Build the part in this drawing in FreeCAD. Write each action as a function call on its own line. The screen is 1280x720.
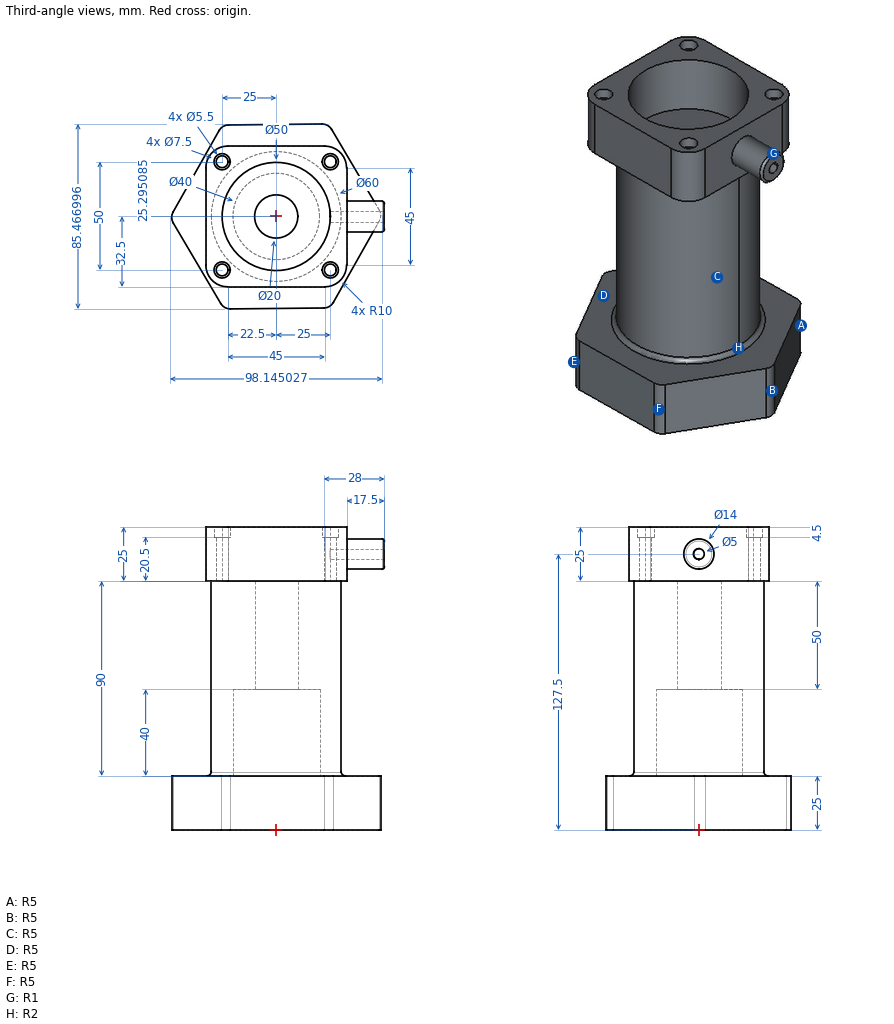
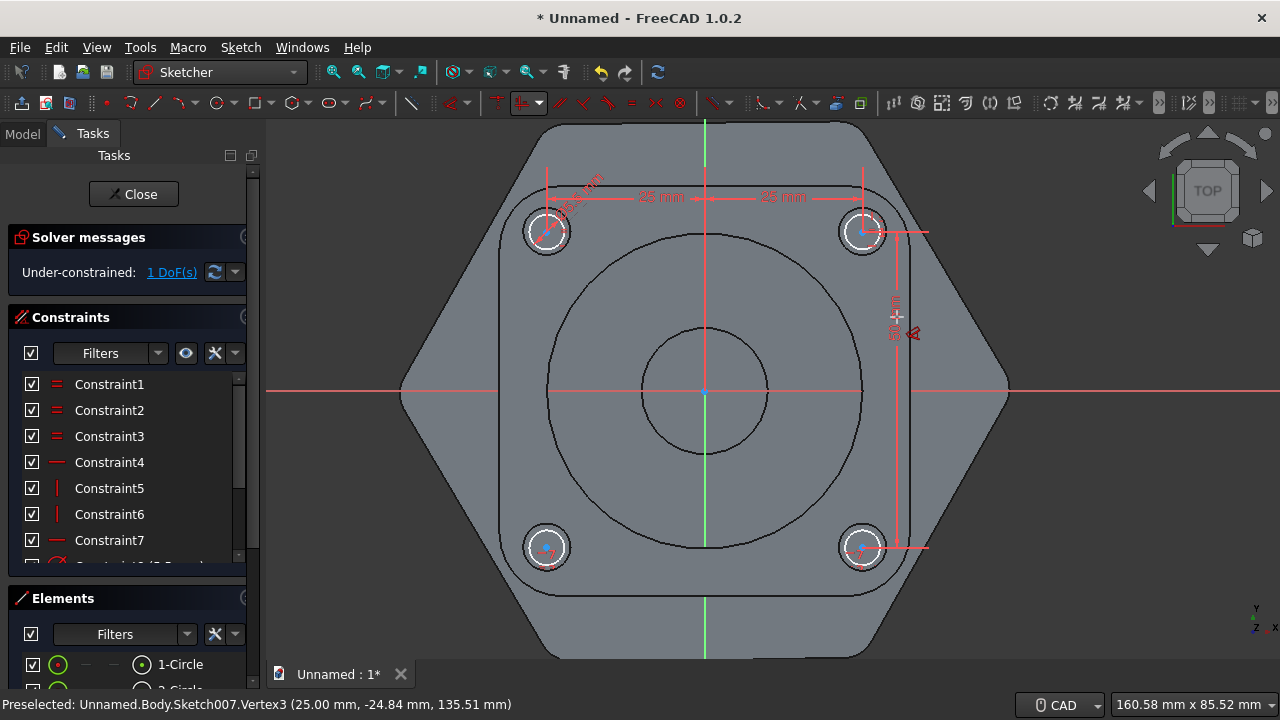
click(547, 232)
click(513, 312)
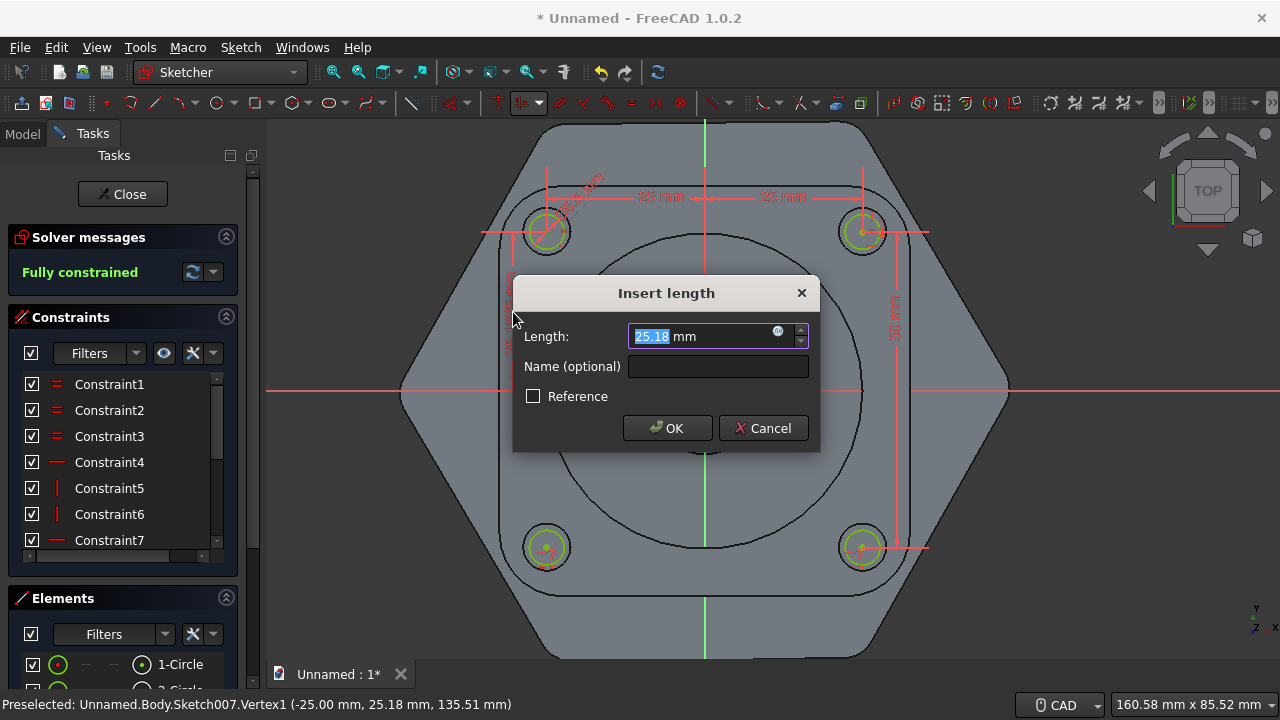
text(25.295085)
key(Return)
key(Escape)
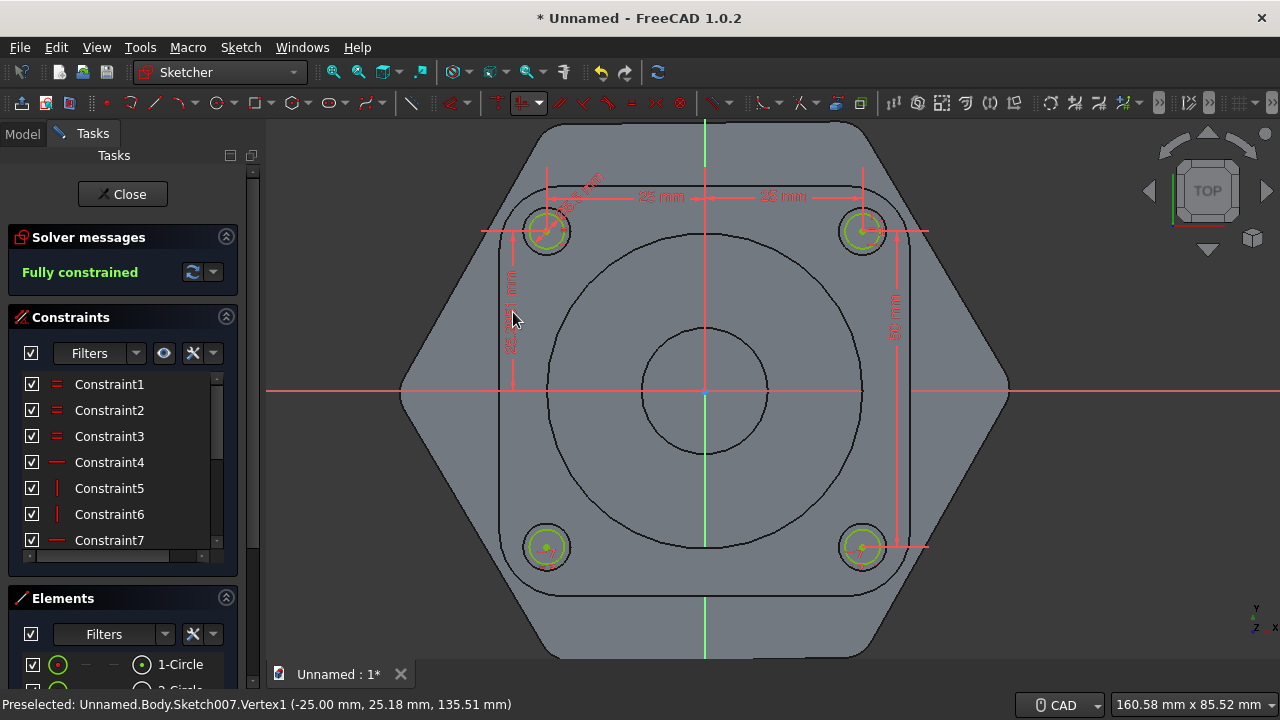
click(123, 194)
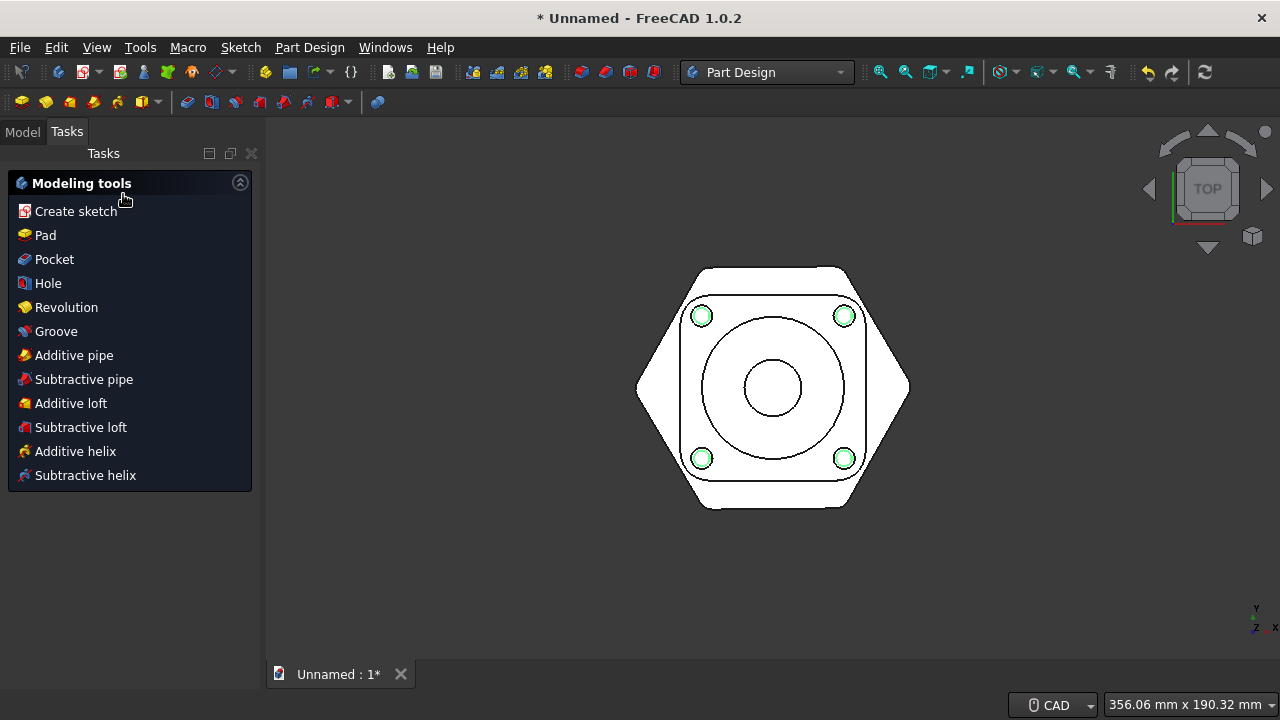
click(188, 102)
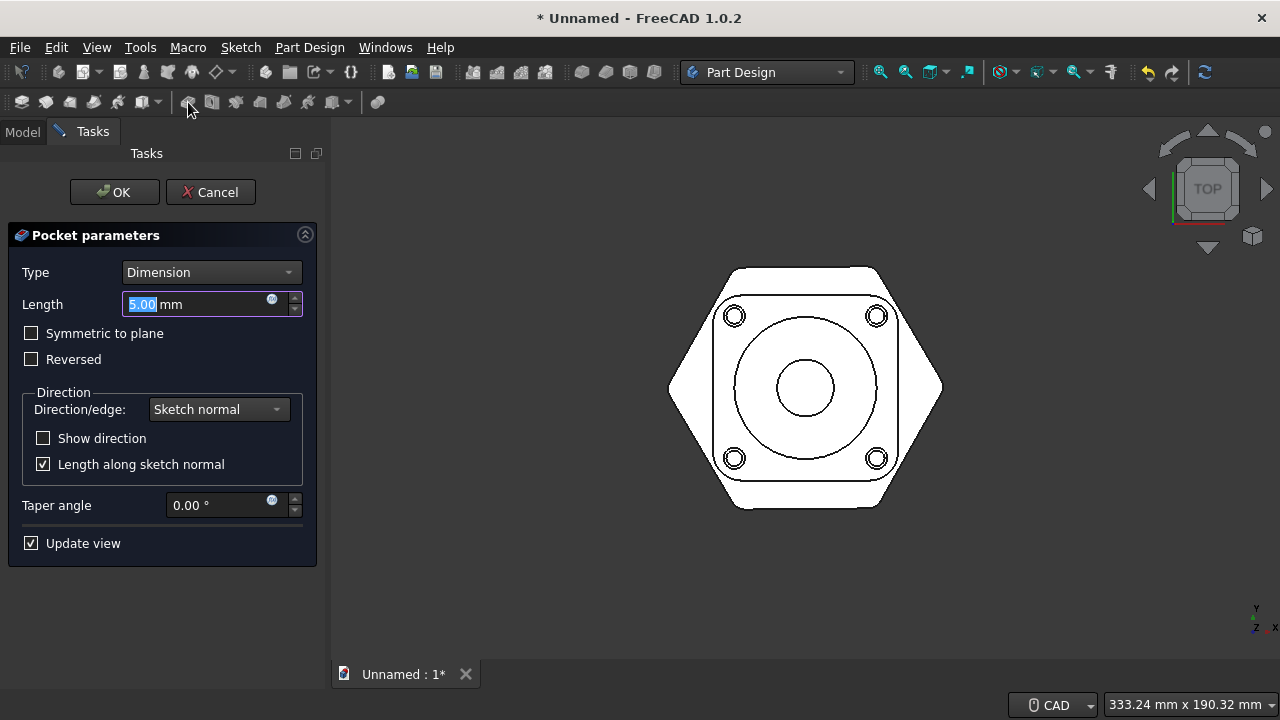
text(20.5)
key(Tab)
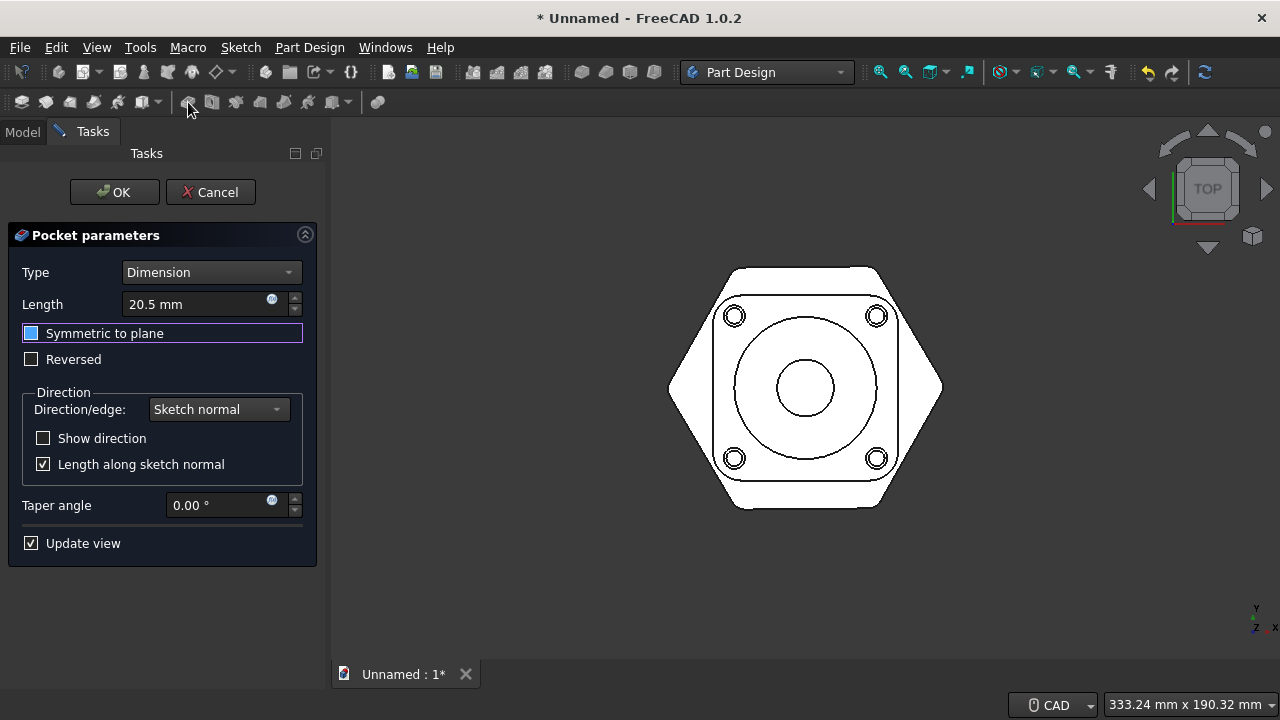
click(115, 192)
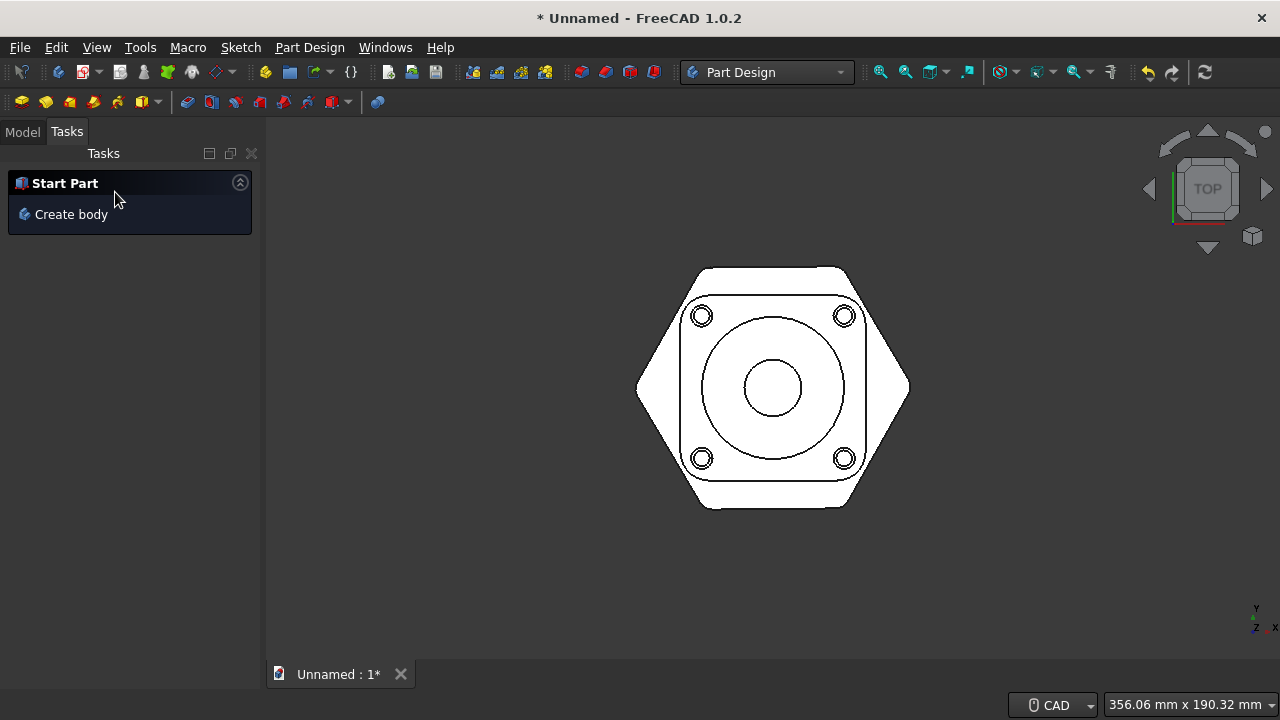
key(0)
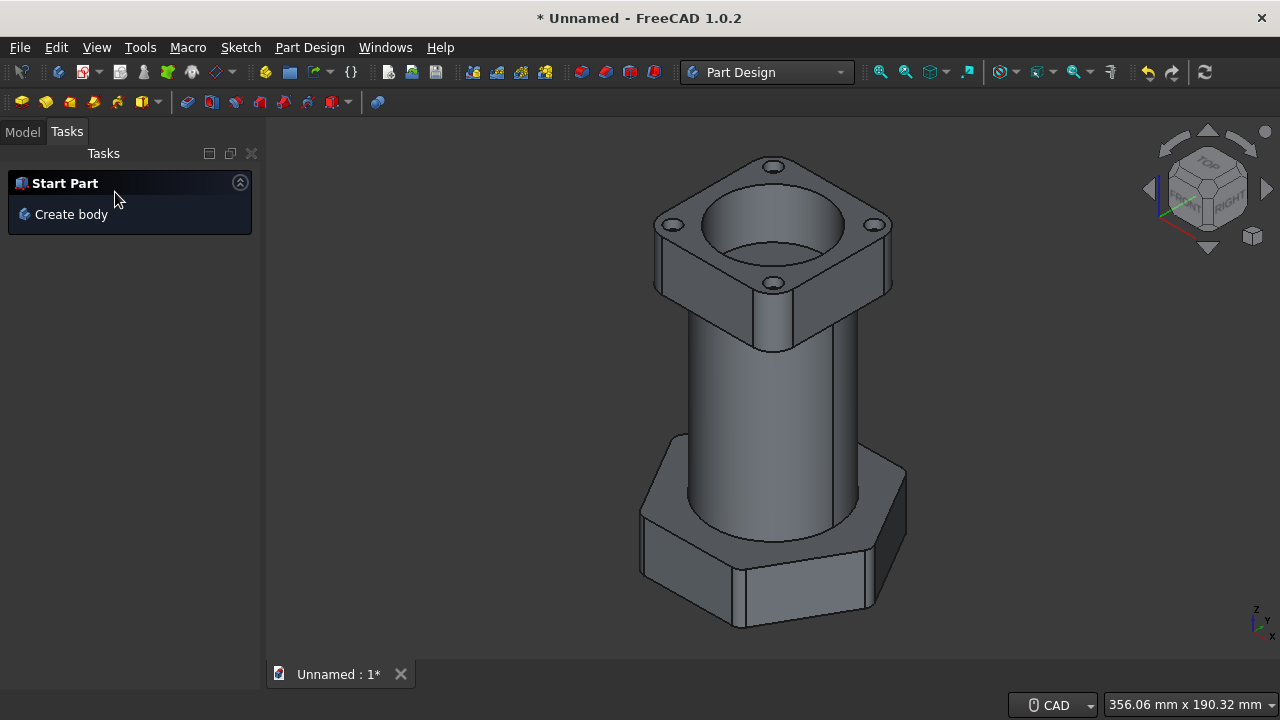
click(851, 284)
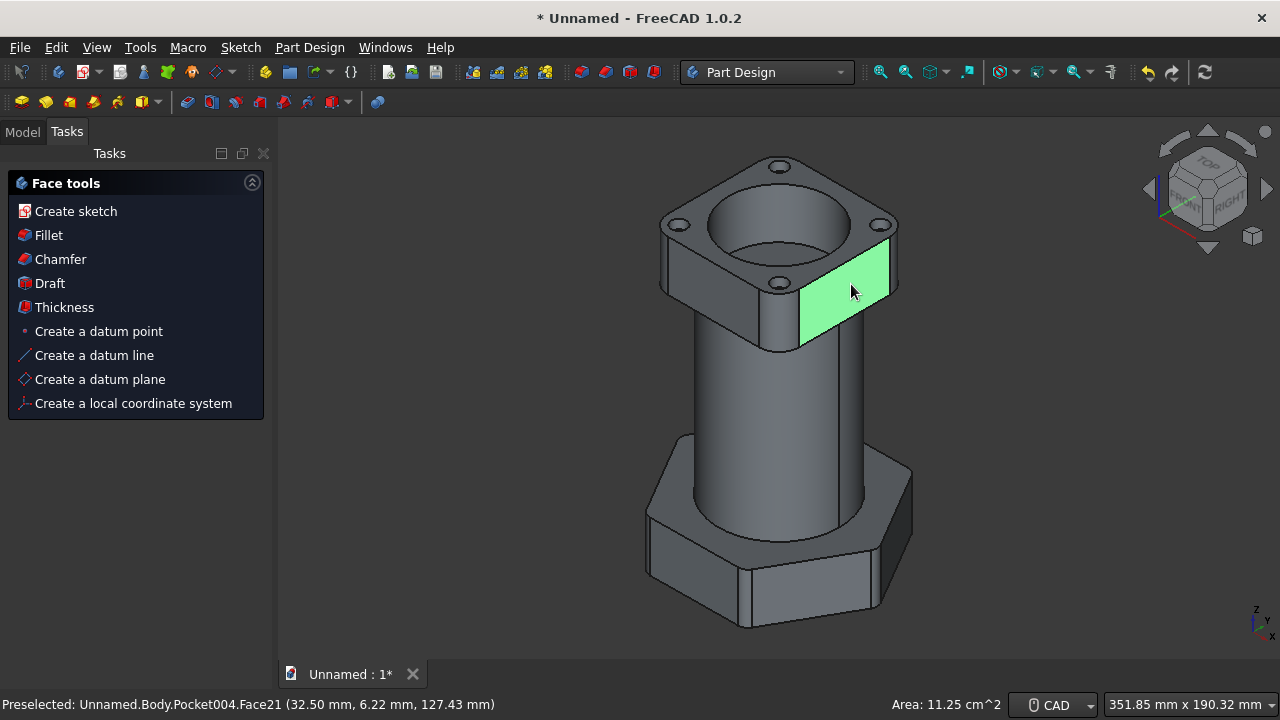
click(84, 72)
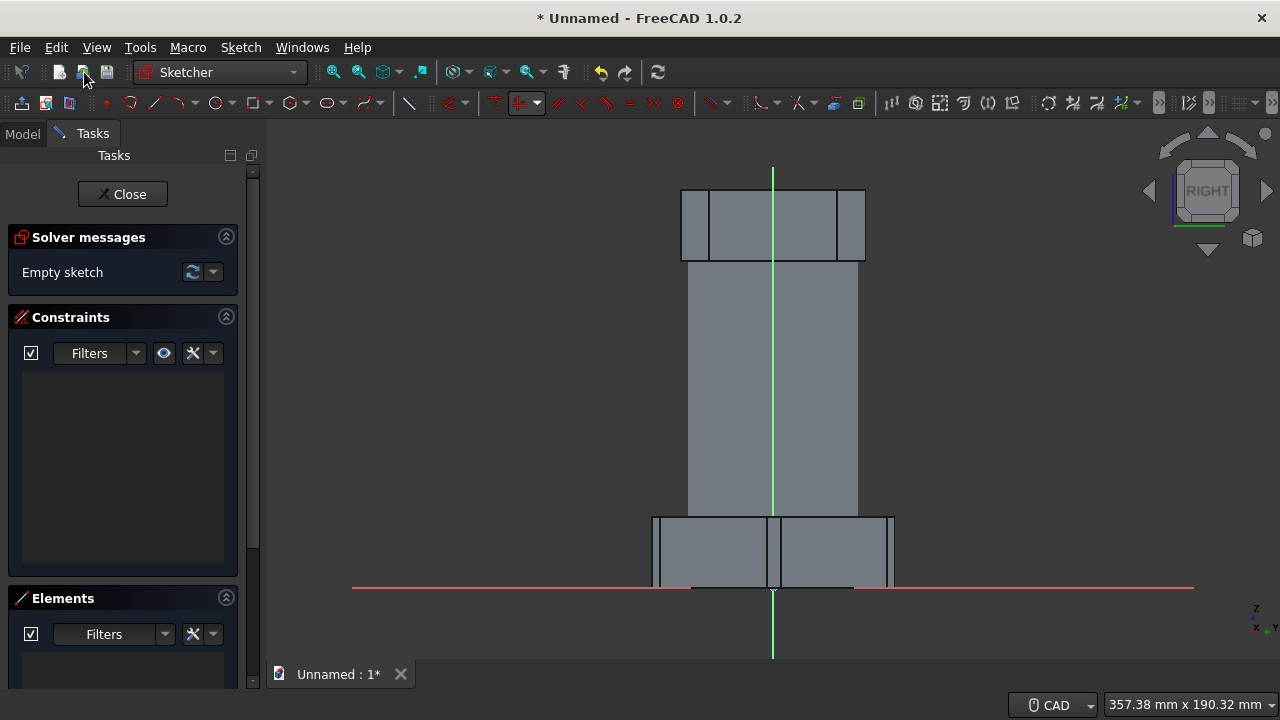
scroll(782, 206, up, 11)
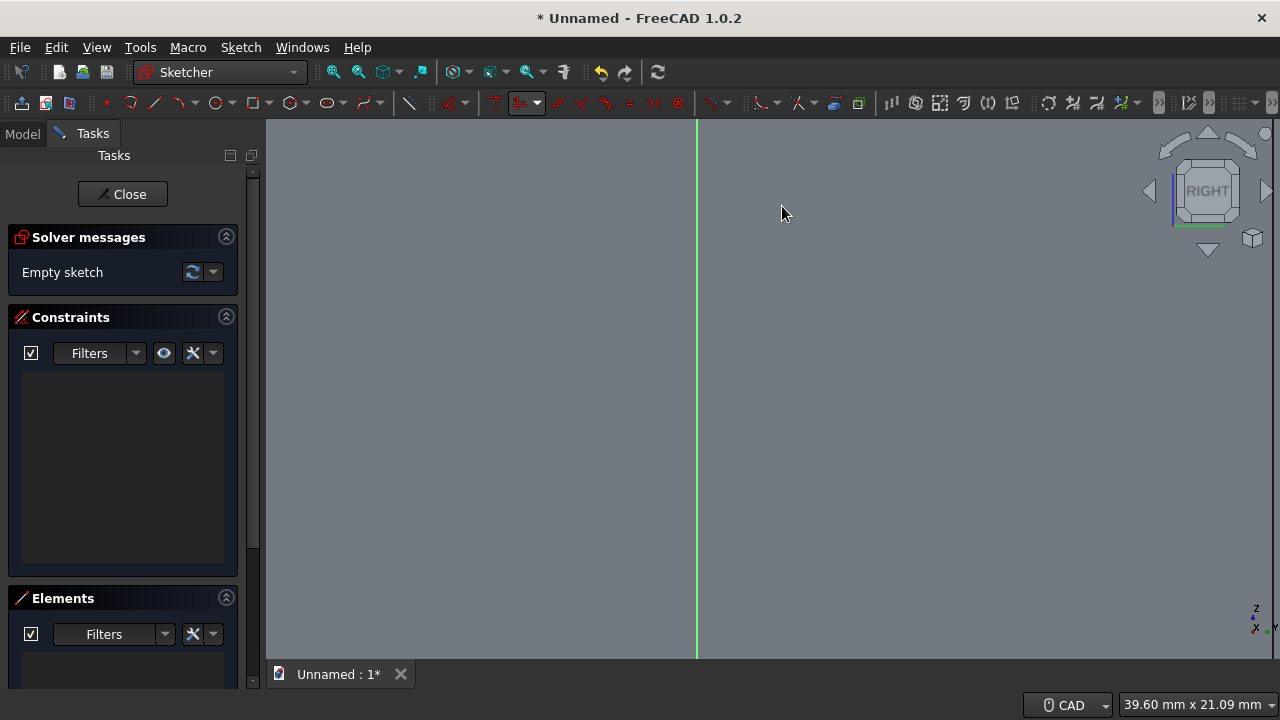
click(216, 104)